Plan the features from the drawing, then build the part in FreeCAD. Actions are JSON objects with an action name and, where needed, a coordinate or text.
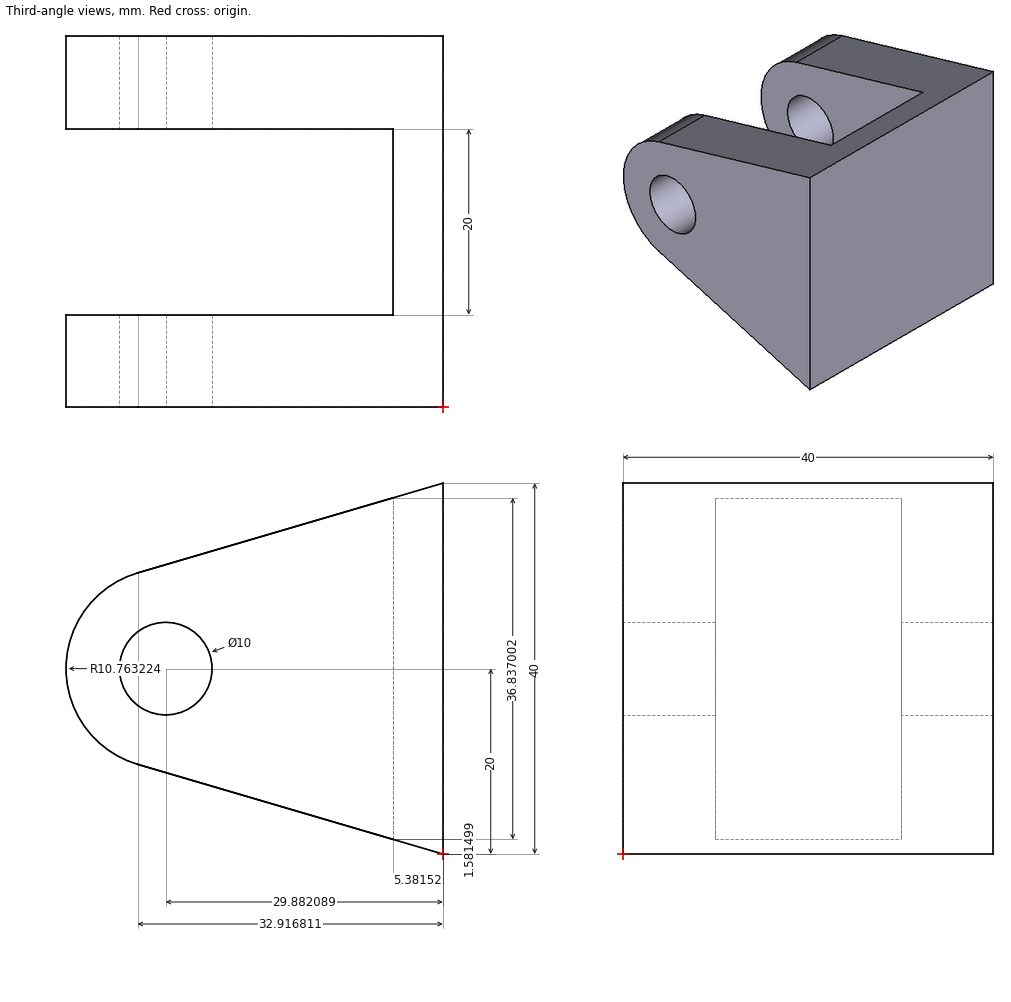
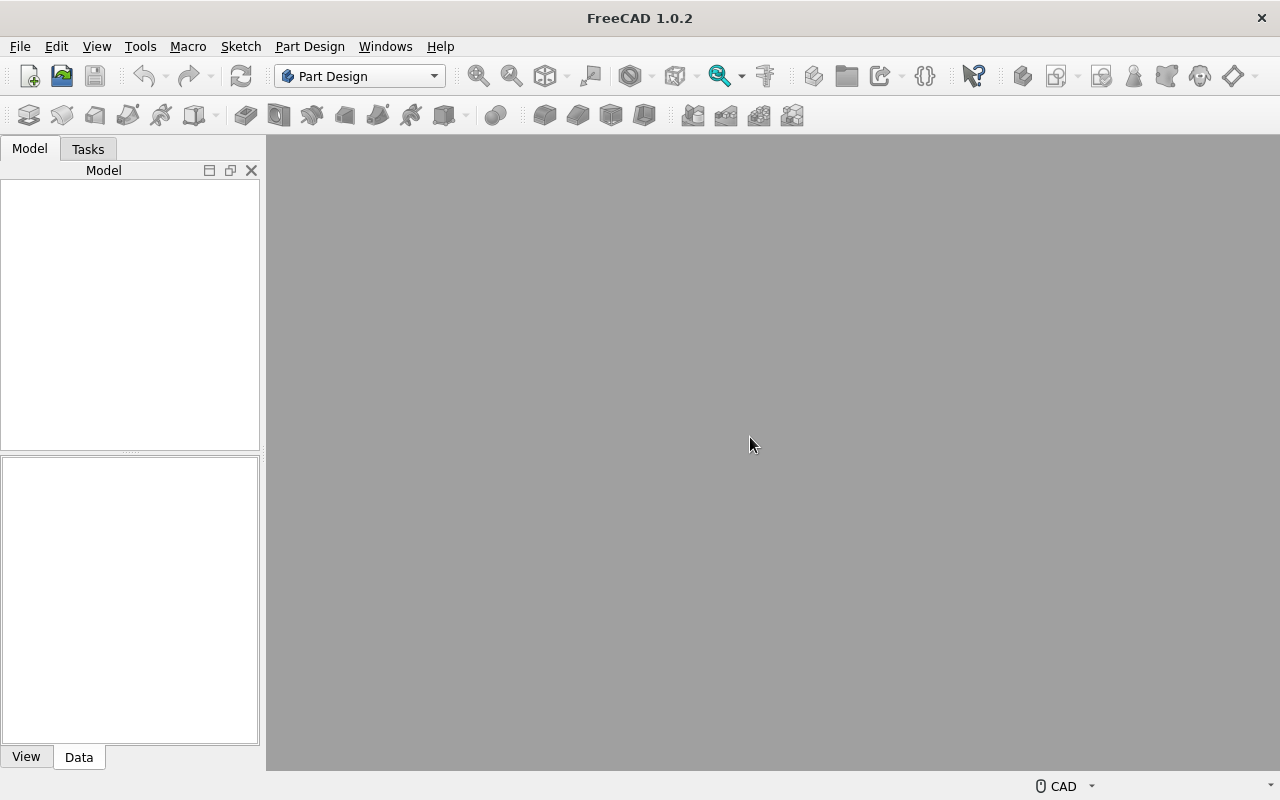
{"action": "left_click", "coordinate": [29, 76]}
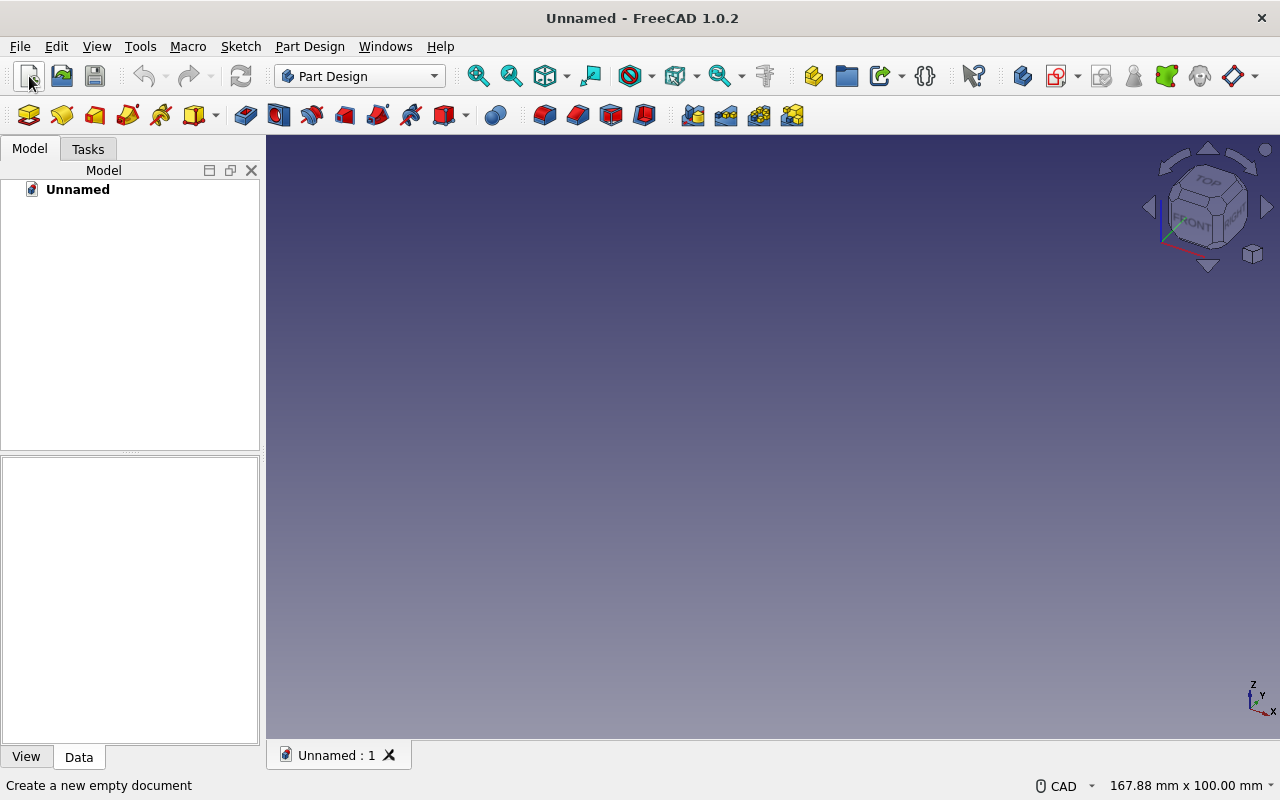
{"action": "left_click", "coordinate": [1056, 76]}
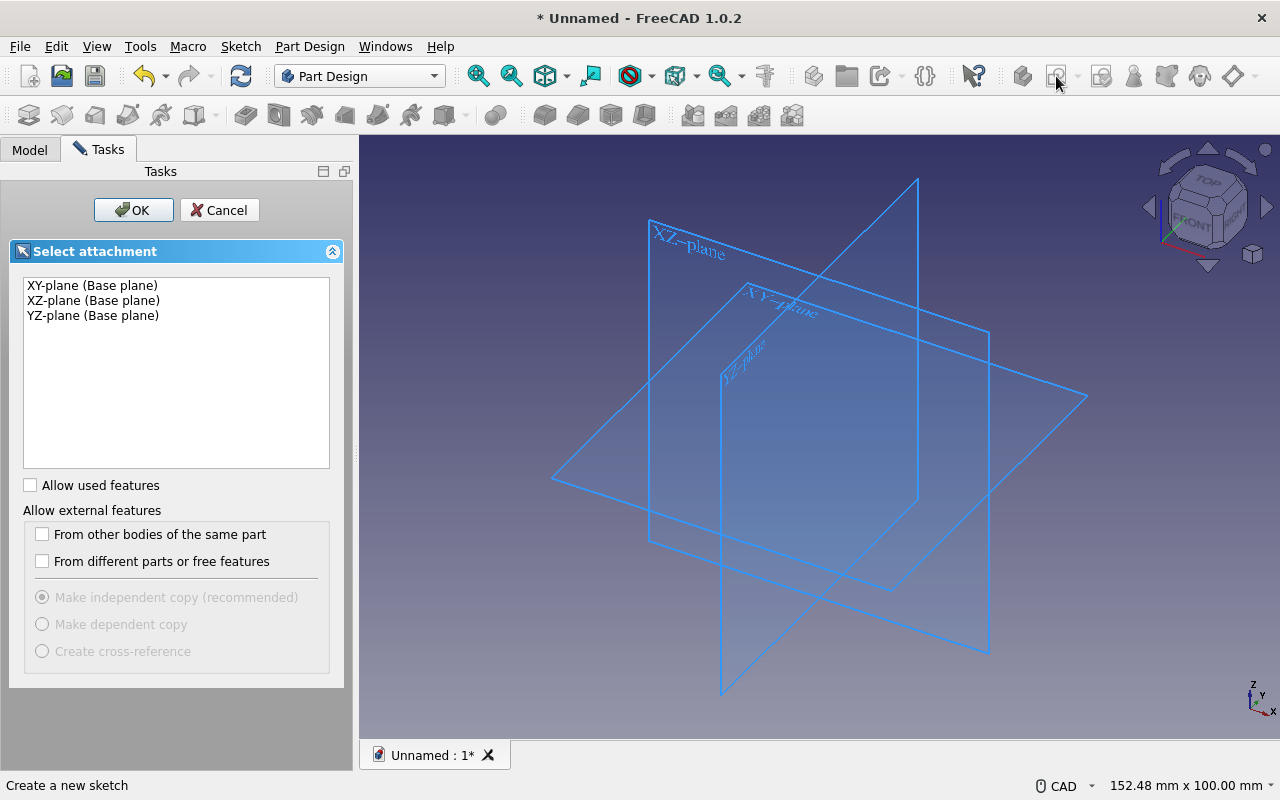
{"action": "left_click", "coordinate": [84, 300]}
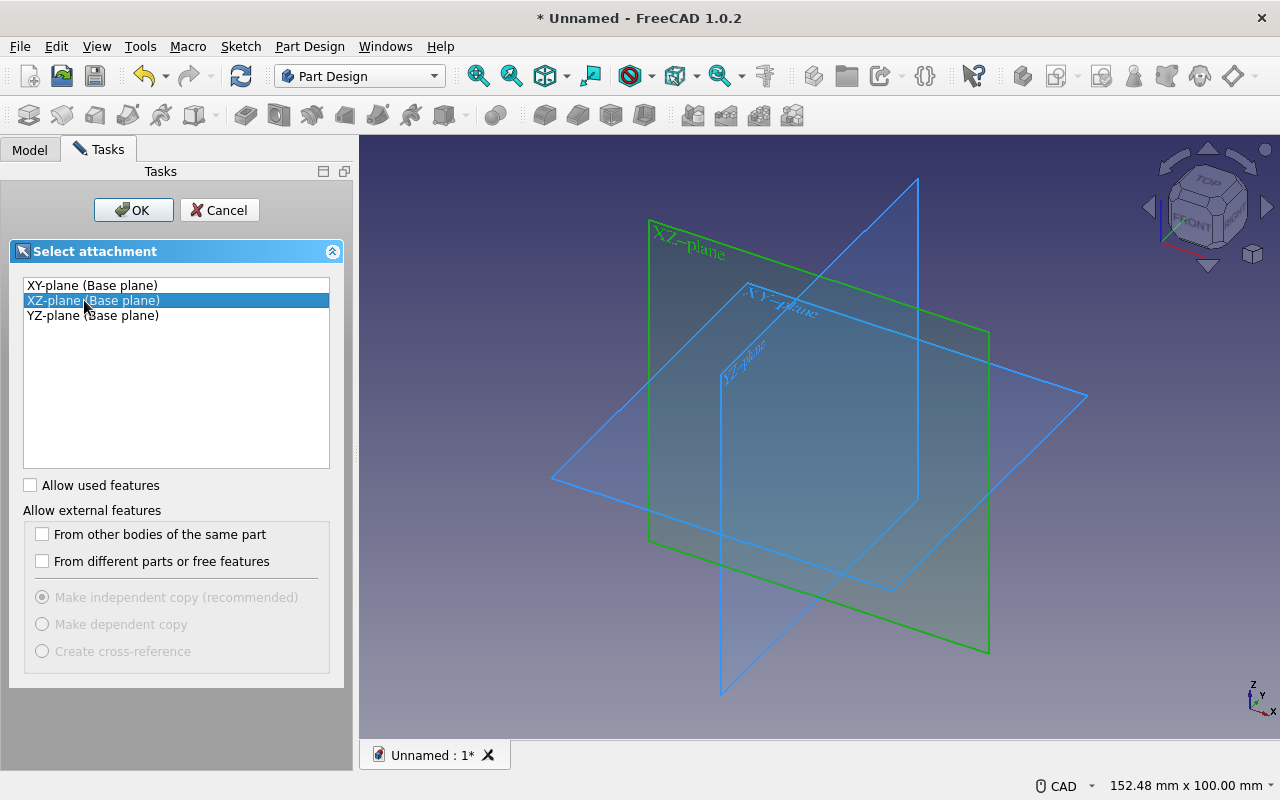
{"action": "left_click", "coordinate": [134, 210]}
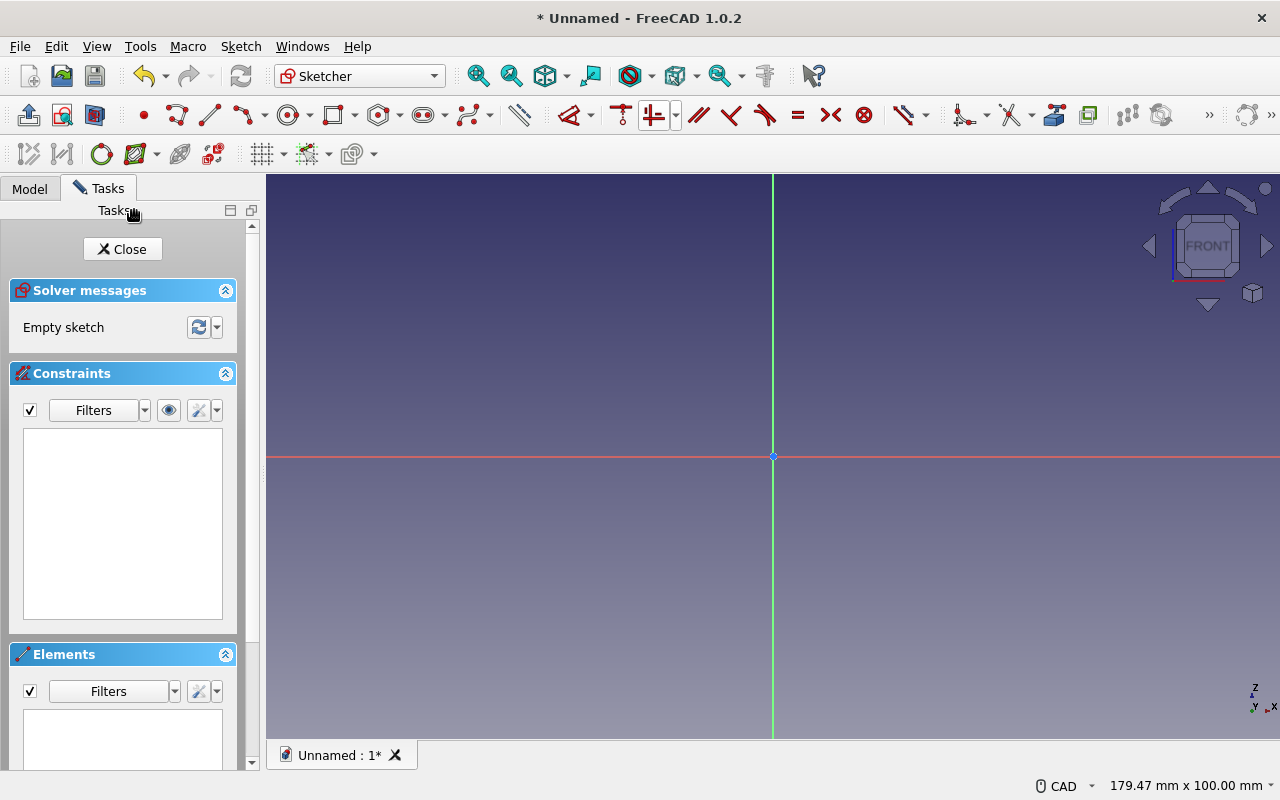
{"action": "scroll", "coordinate": [564, 202], "scroll_direction": "up", "scroll_amount": 2}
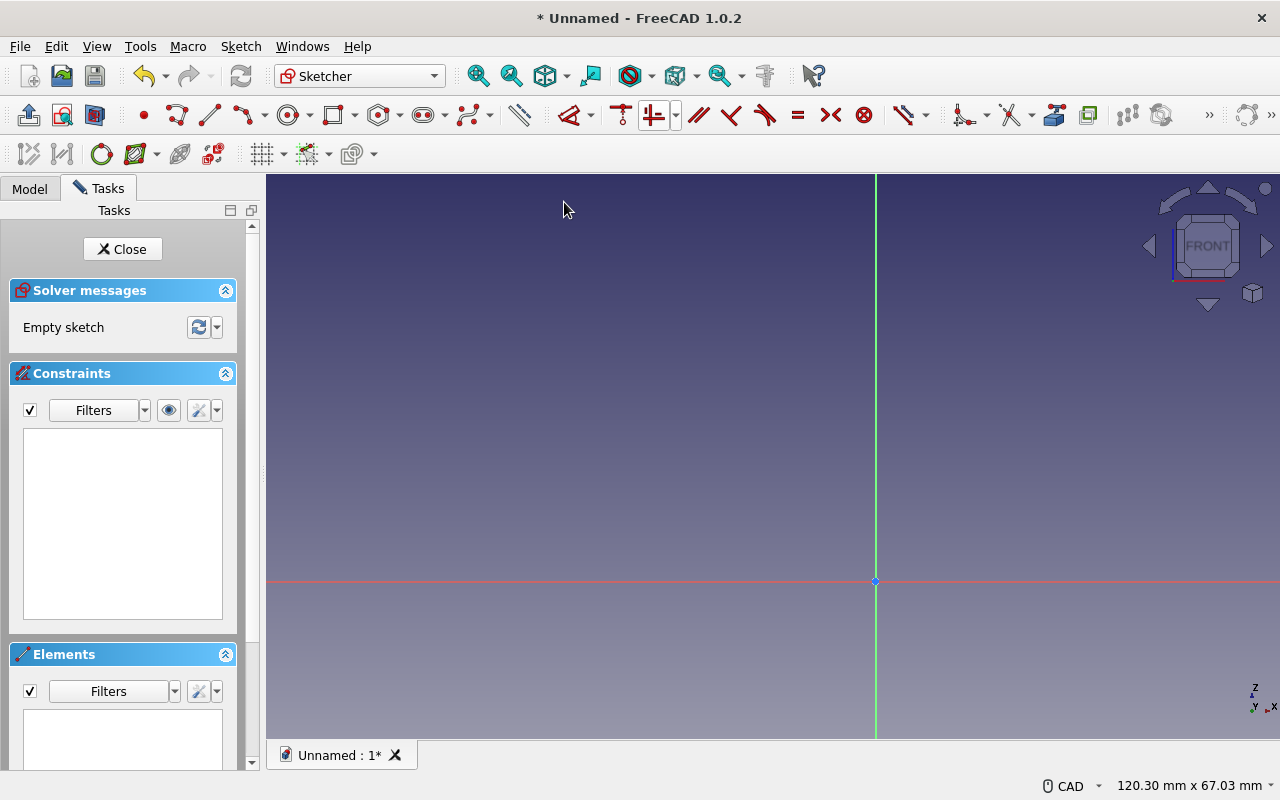
{"action": "left_click", "coordinate": [177, 116]}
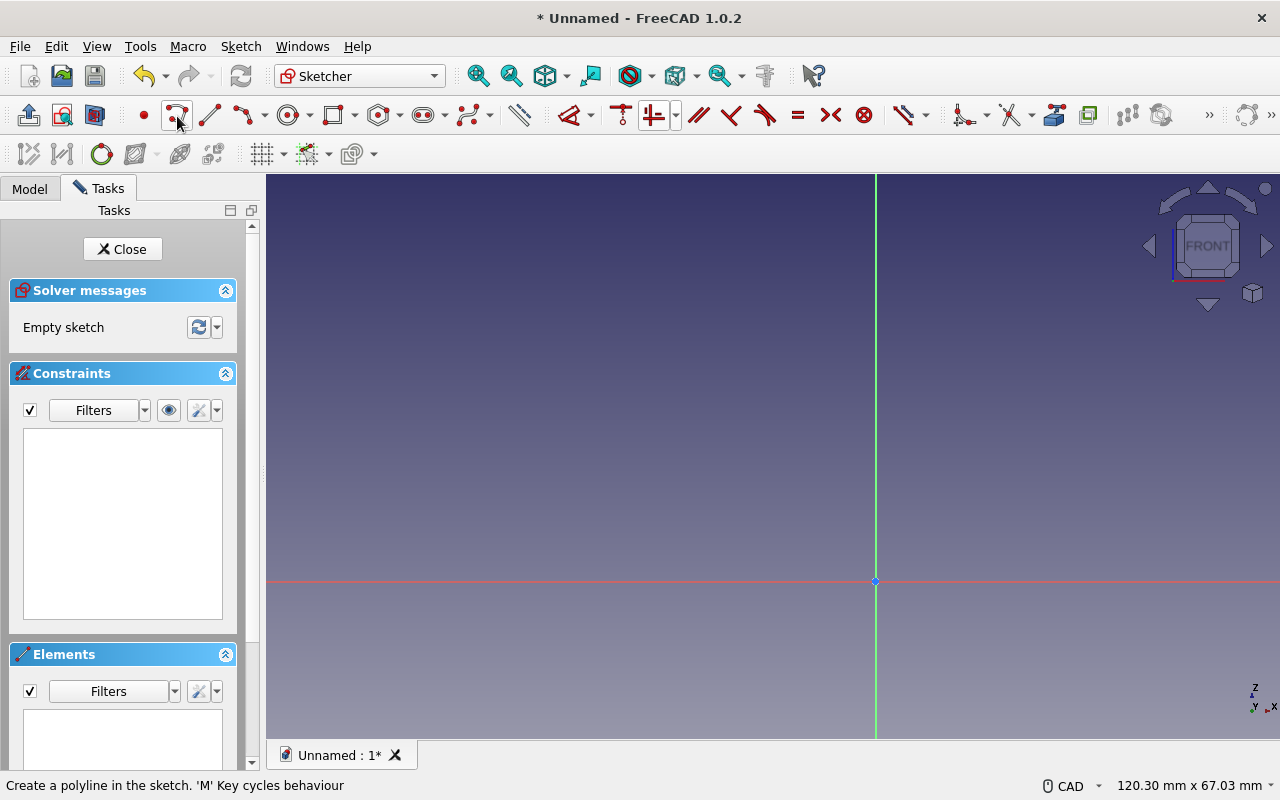
{"action": "left_click", "coordinate": [598, 326]}
{"action": "left_click", "coordinate": [876, 244]}
{"action": "left_click", "coordinate": [876, 582]}
{"action": "left_click", "coordinate": [598, 500]}
{"action": "right_click", "coordinate": [598, 500]}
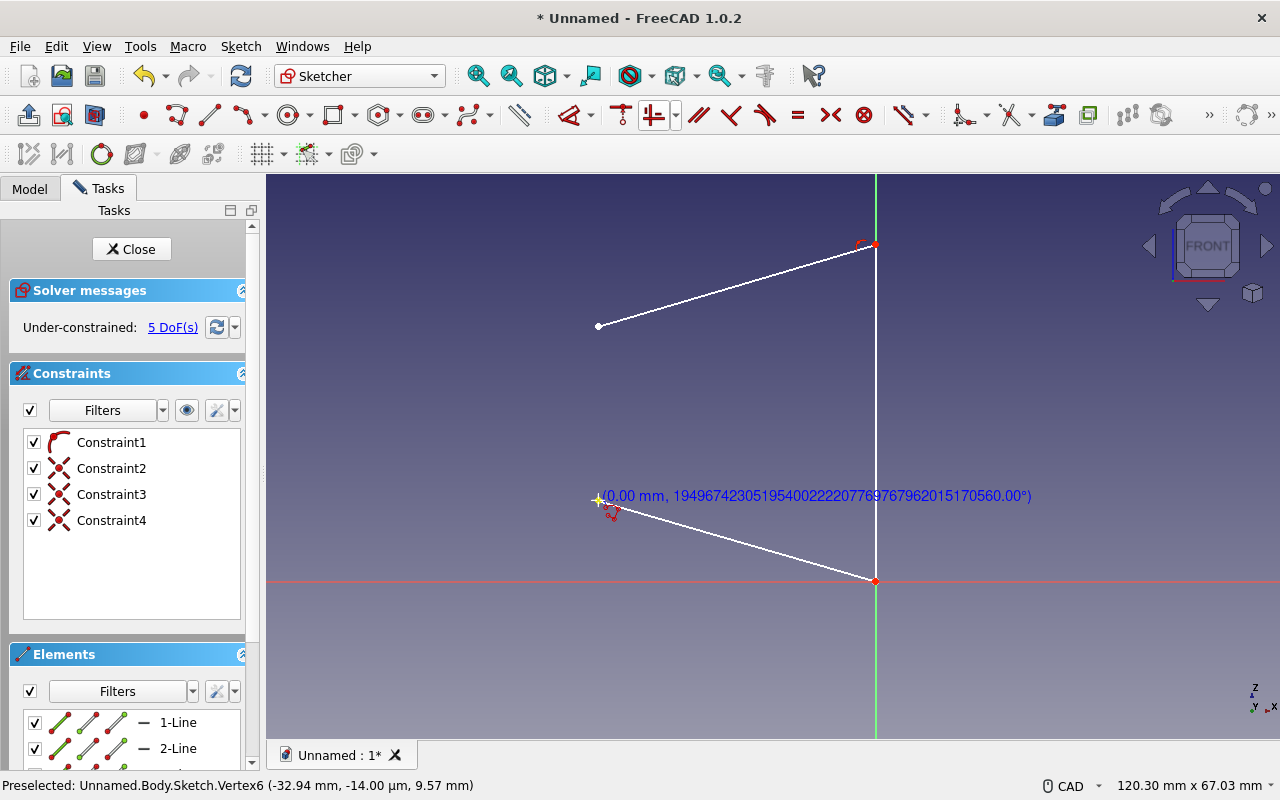
{"action": "left_click", "coordinate": [242, 116]}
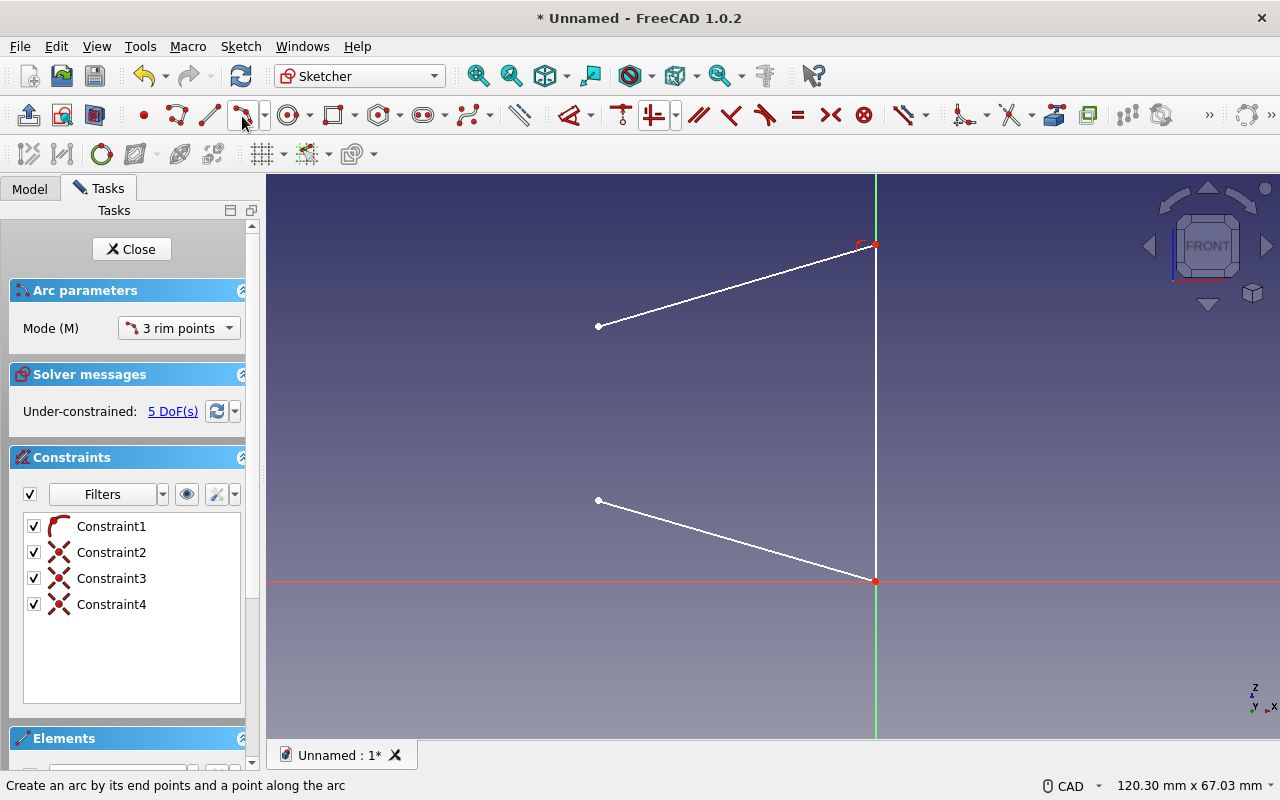
{"action": "left_click", "coordinate": [598, 501]}
{"action": "left_click", "coordinate": [598, 327]}
{"action": "left_click", "coordinate": [533, 413]}
{"action": "key", "text": "Escape"}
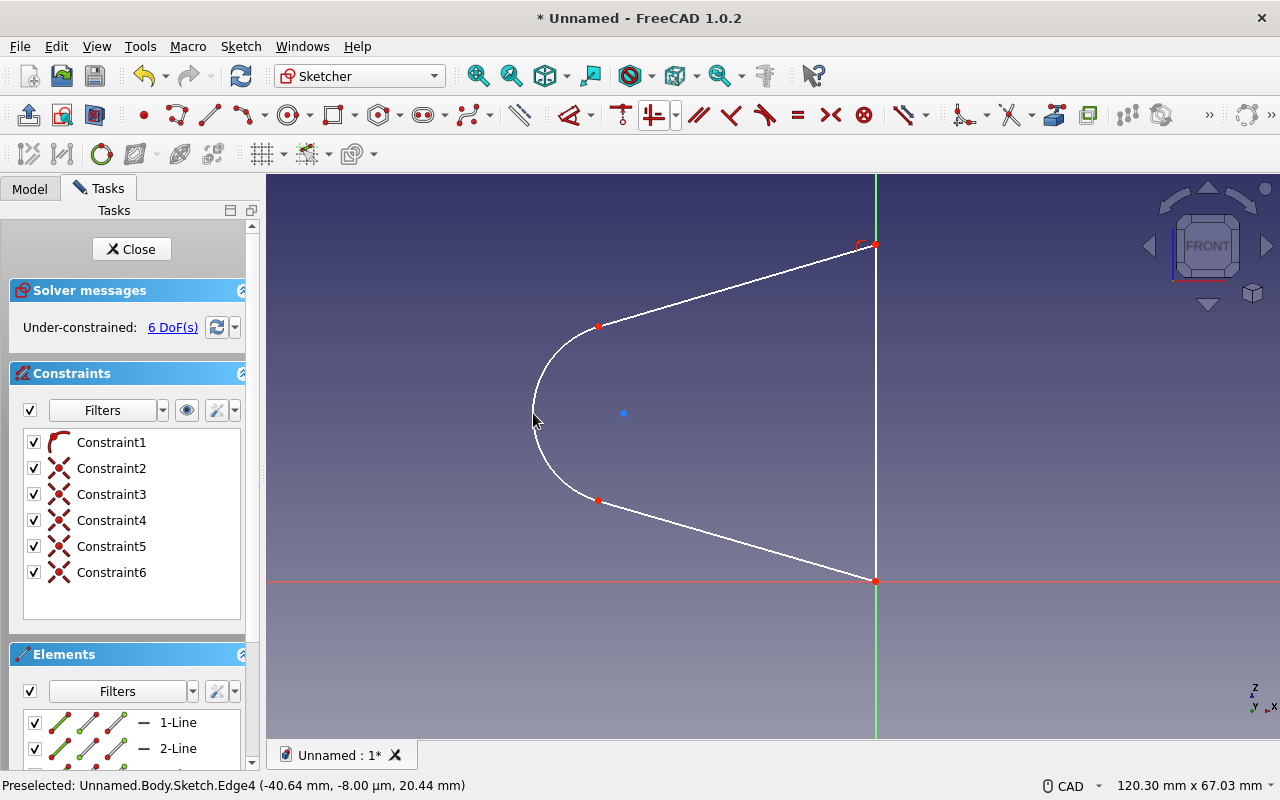
{"action": "left_click", "coordinate": [681, 302]}